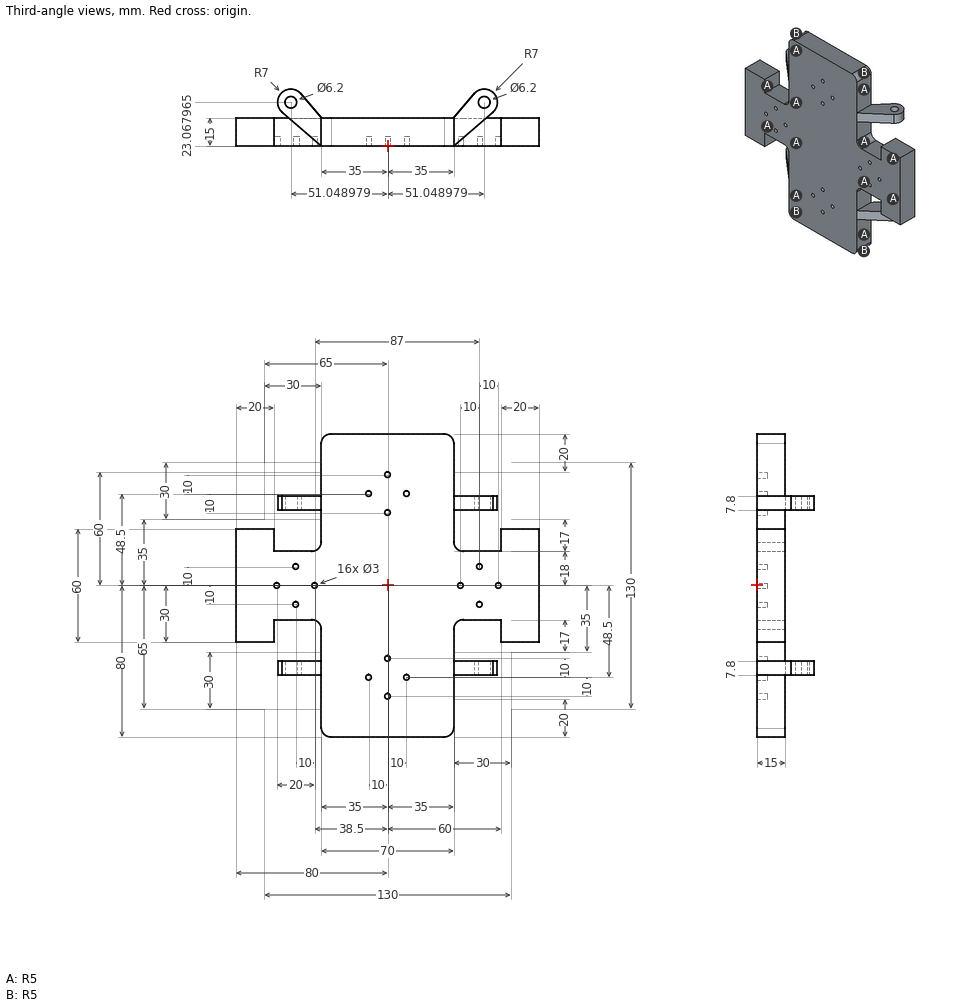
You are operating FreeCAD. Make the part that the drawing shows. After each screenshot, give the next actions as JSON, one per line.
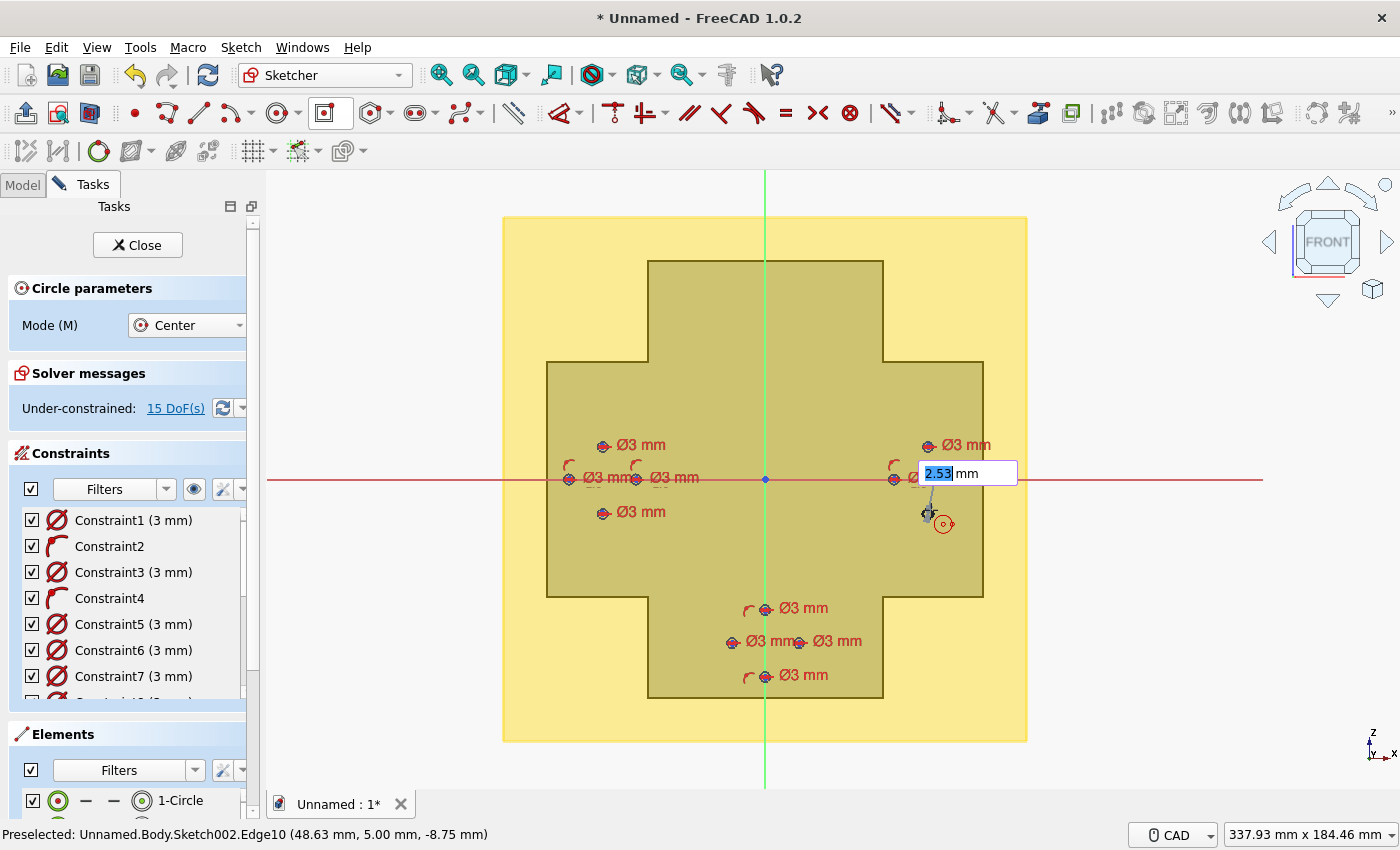
{"action": "type", "text": "3"}
{"action": "key", "text": "Return"}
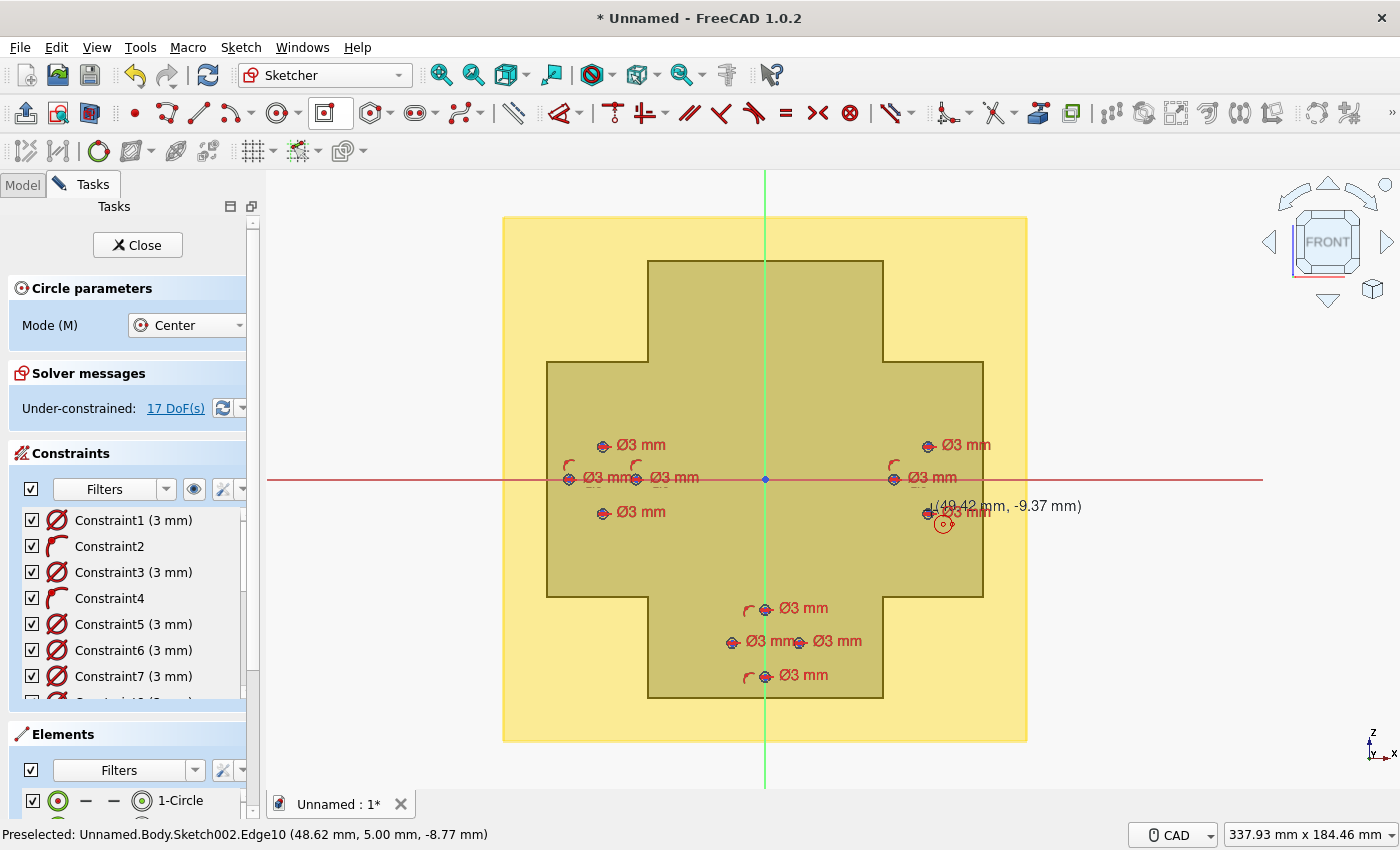
{"action": "scroll", "coordinate": [961, 480], "scroll_direction": "up", "scroll_amount": 8}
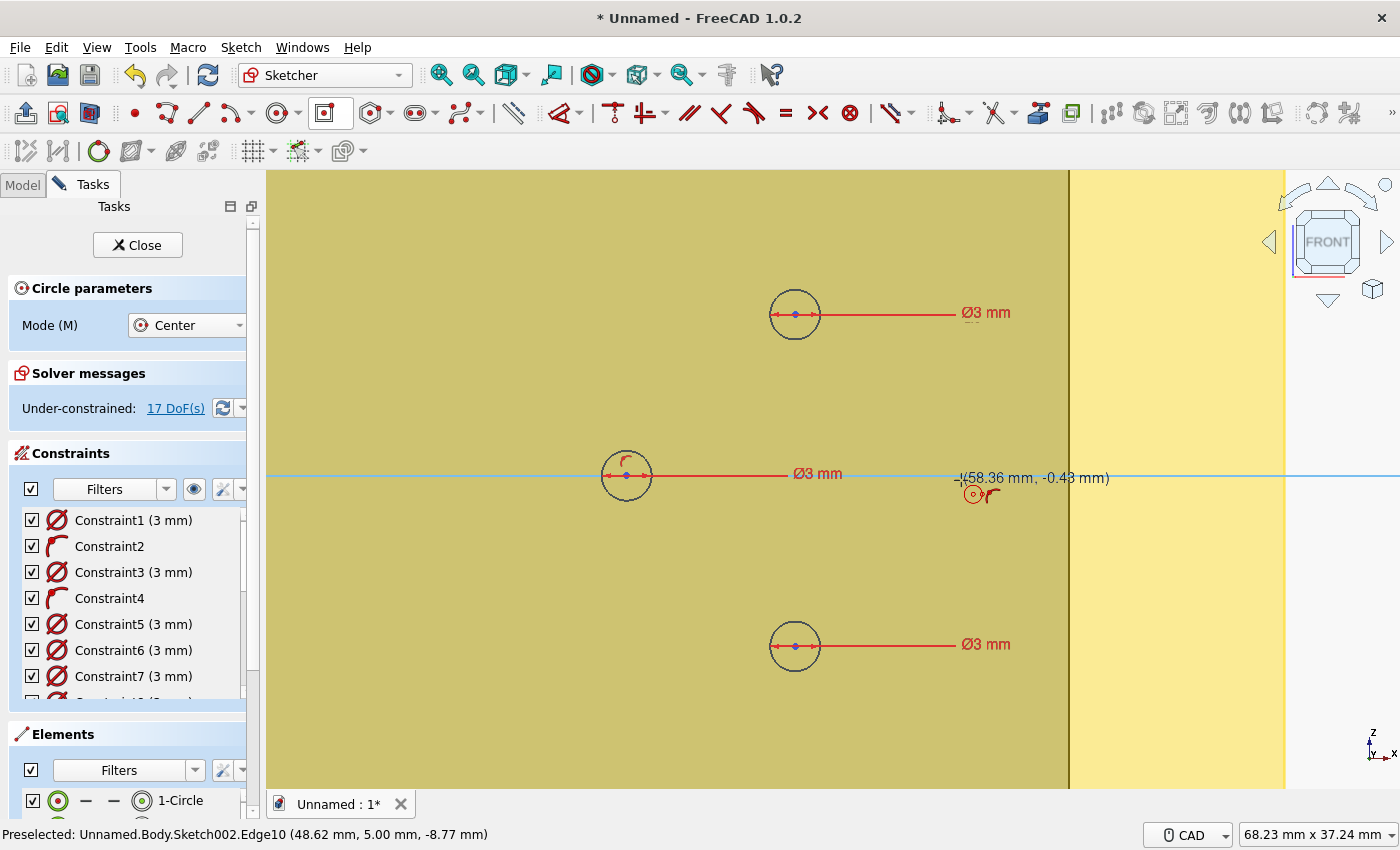
{"action": "scroll", "coordinate": [961, 480], "scroll_direction": "down", "scroll_amount": 8}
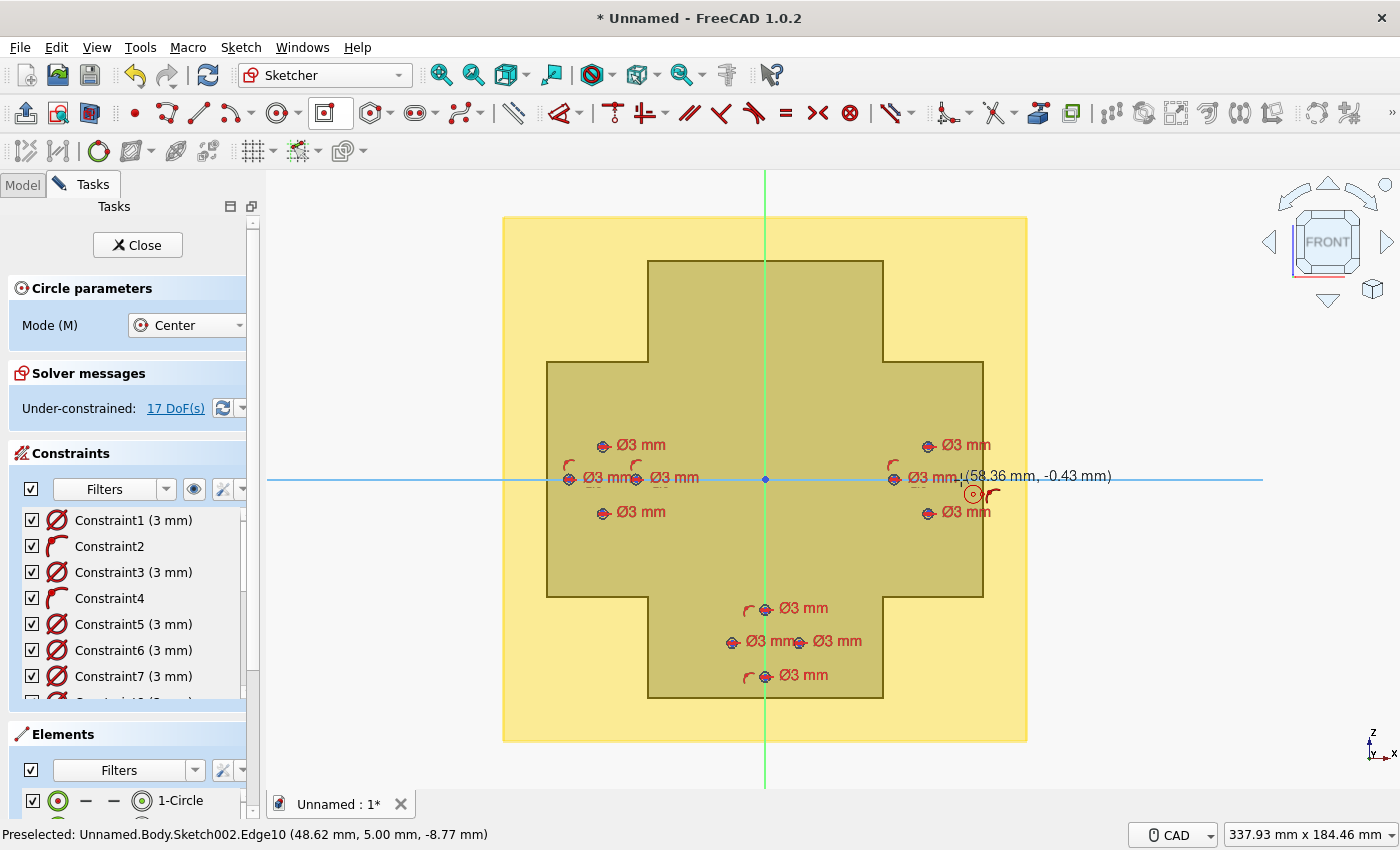
{"action": "left_click", "coordinate": [961, 480]}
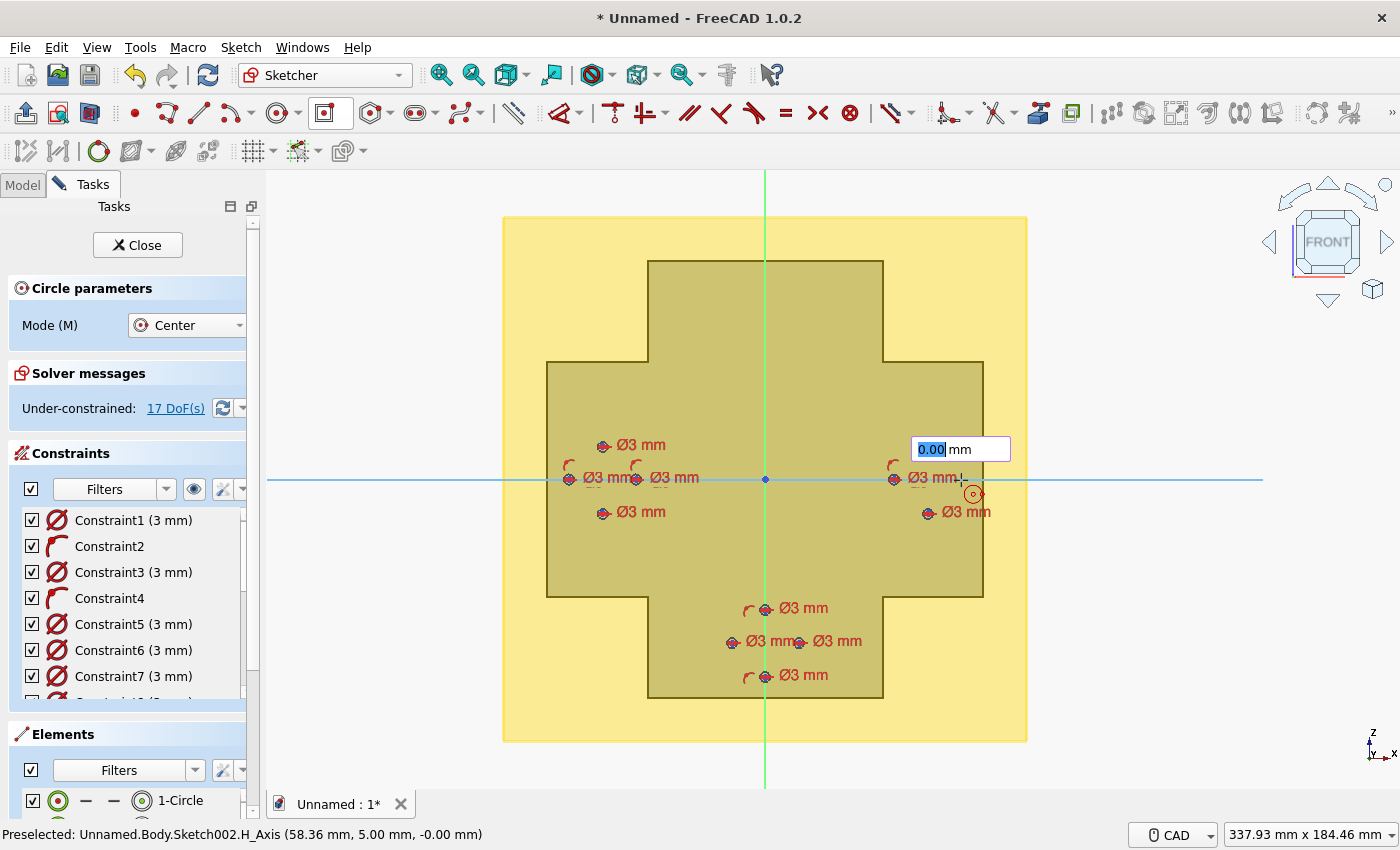
{"action": "scroll", "coordinate": [960, 484], "scroll_direction": "up", "scroll_amount": 7}
{"action": "mouse_move", "coordinate": [957, 484]}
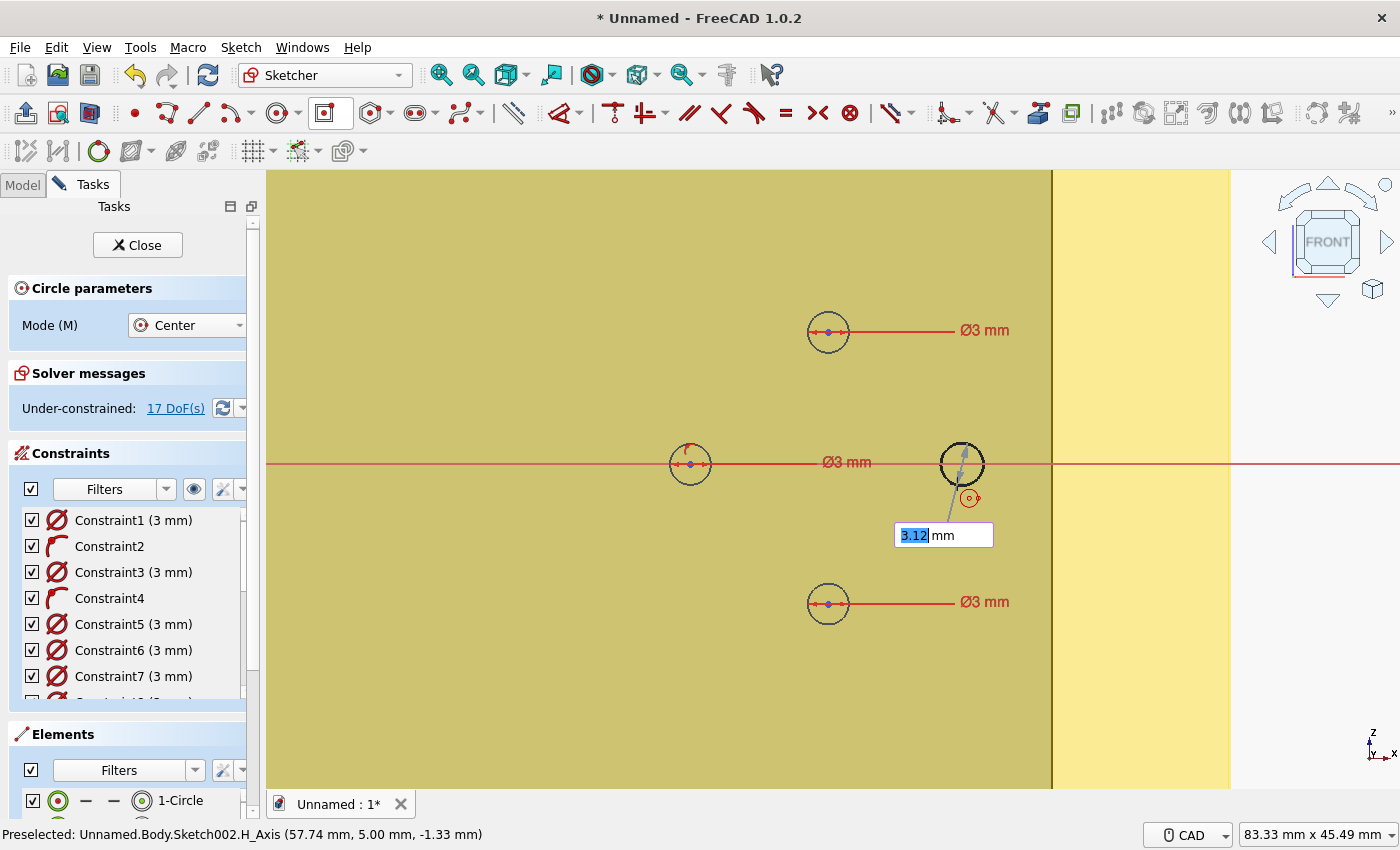
{"action": "type", "text": "3"}
{"action": "key", "text": "Return"}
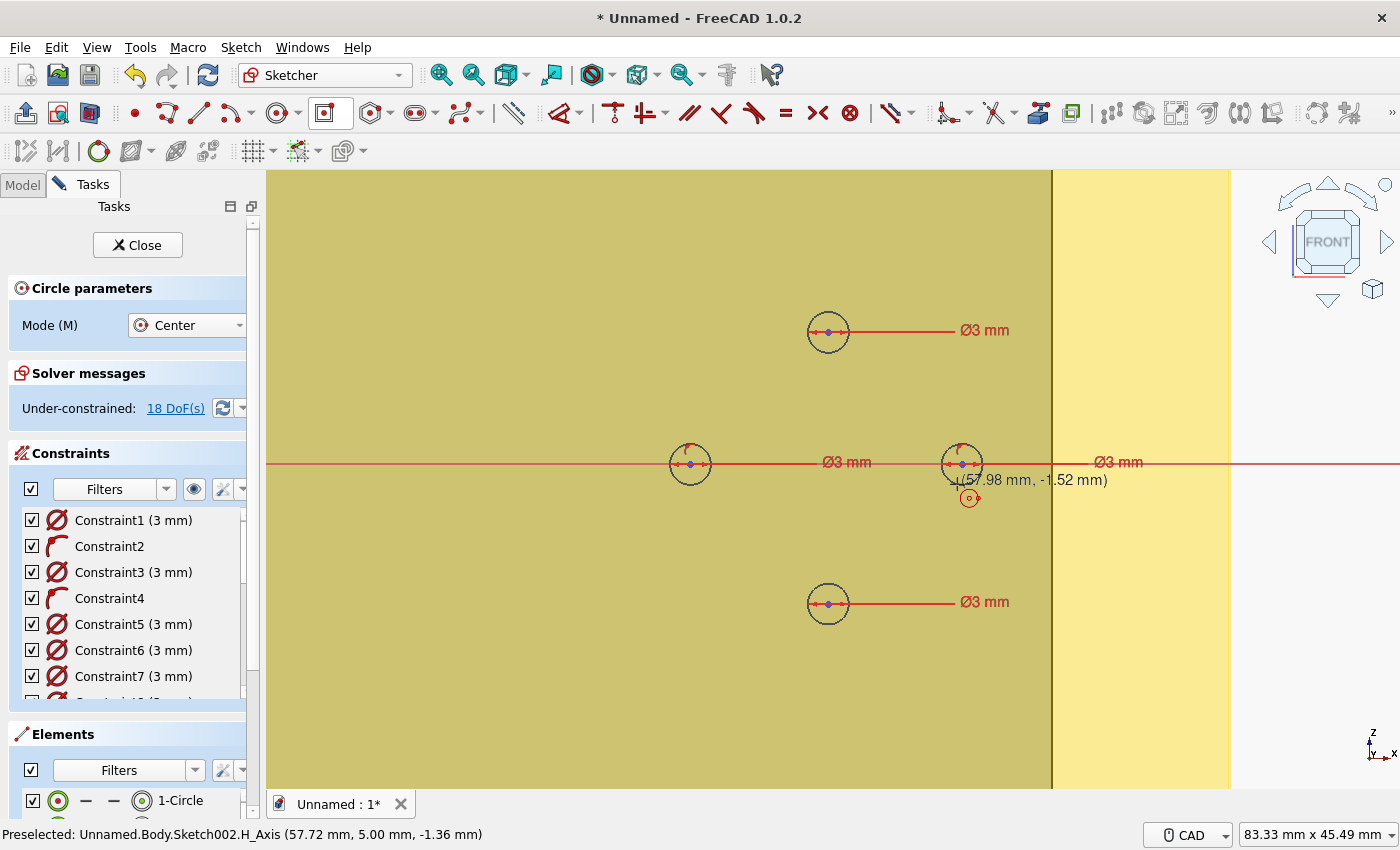
{"action": "scroll", "coordinate": [960, 484], "scroll_direction": "down", "scroll_amount": 7}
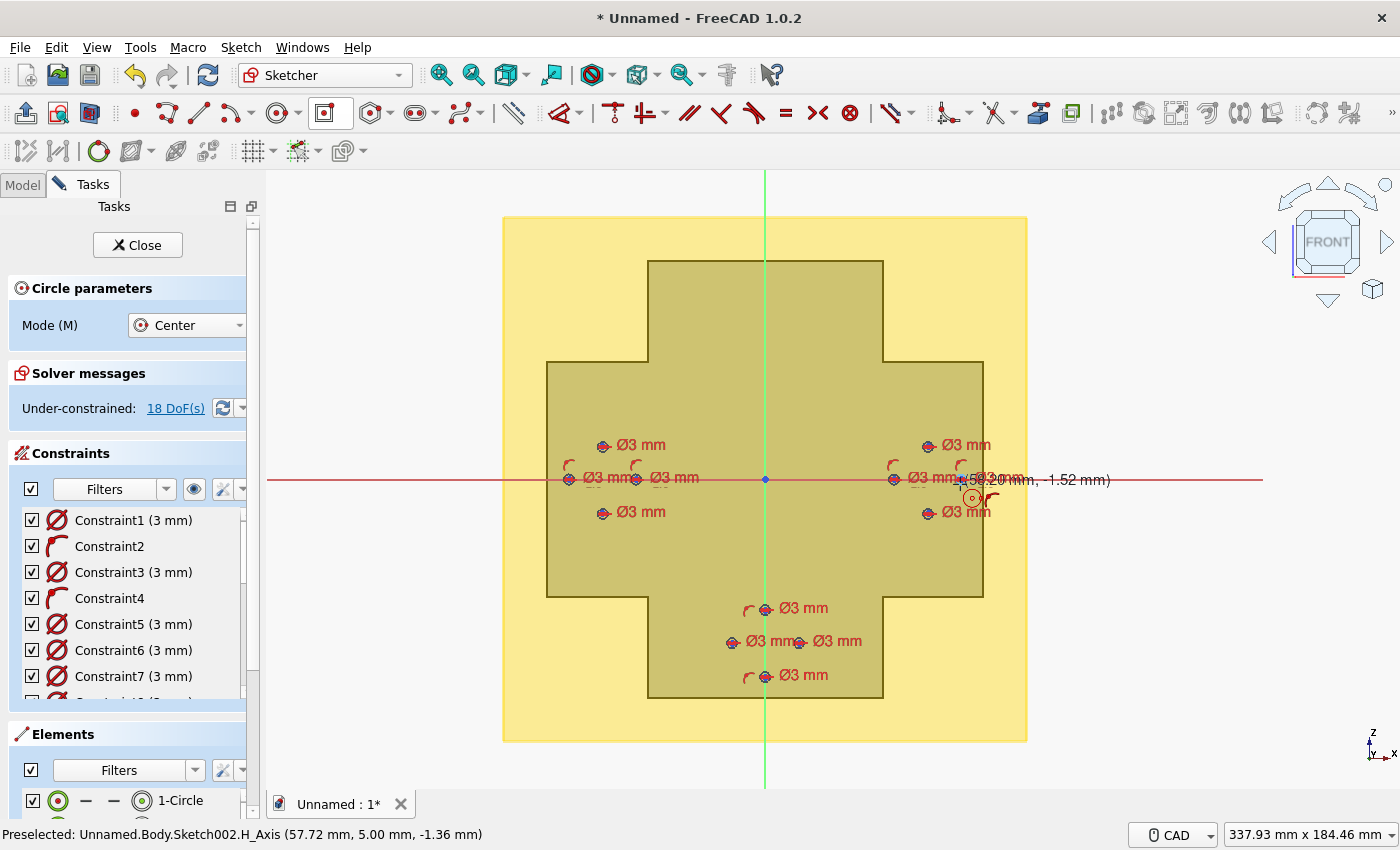
{"action": "scroll", "coordinate": [732, 317], "scroll_direction": "up", "scroll_amount": 8}